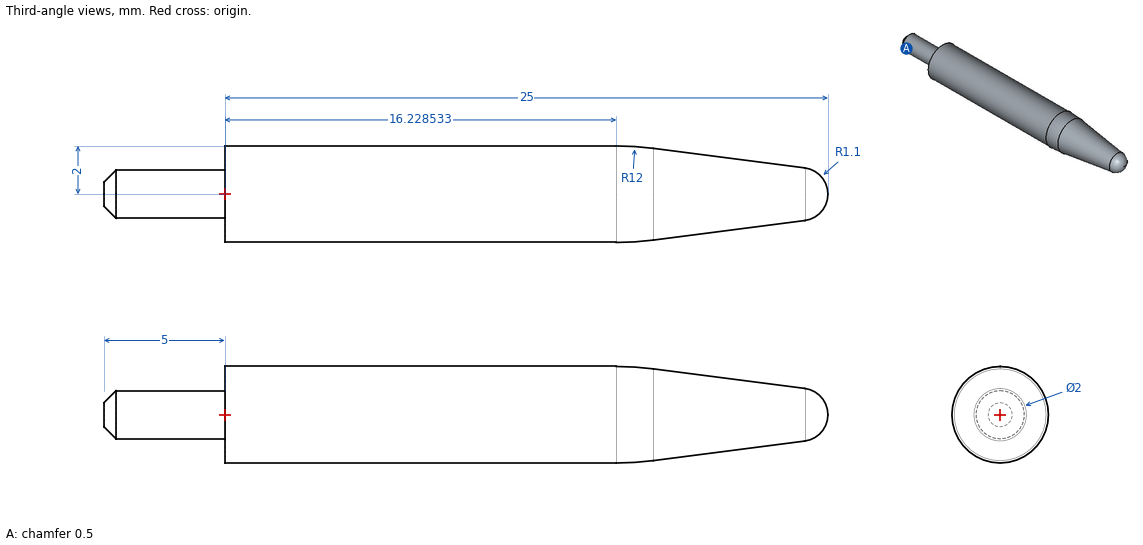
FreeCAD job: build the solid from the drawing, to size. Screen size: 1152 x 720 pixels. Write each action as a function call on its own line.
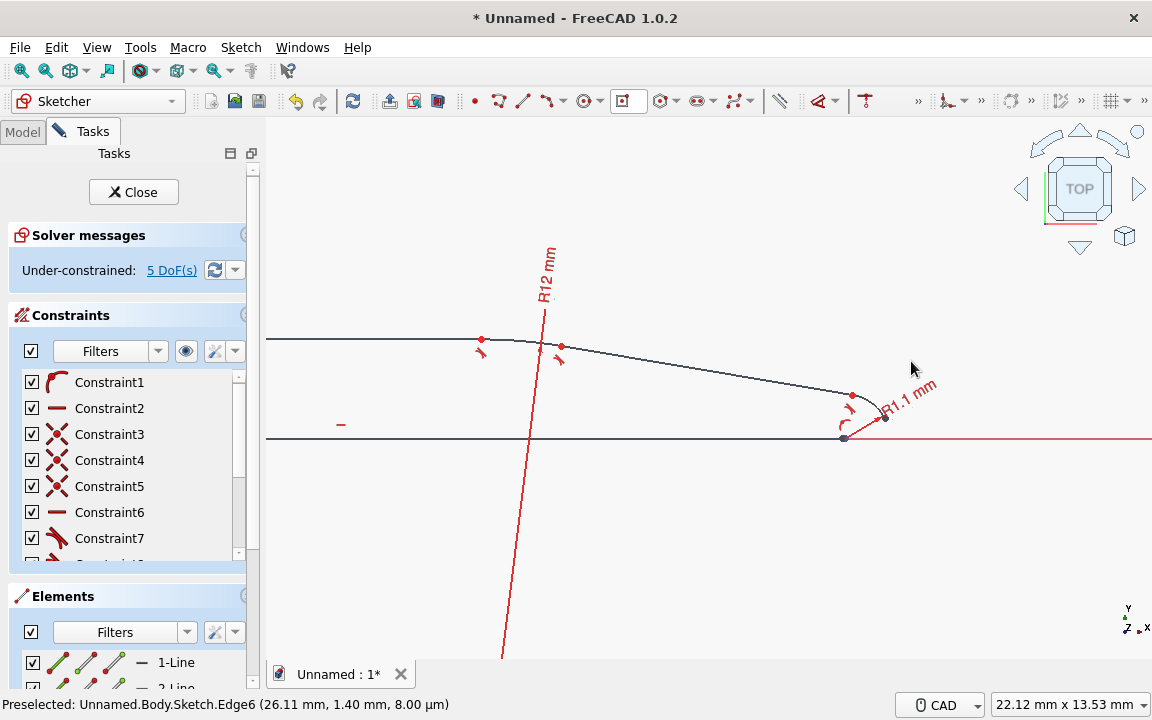
click(885, 419)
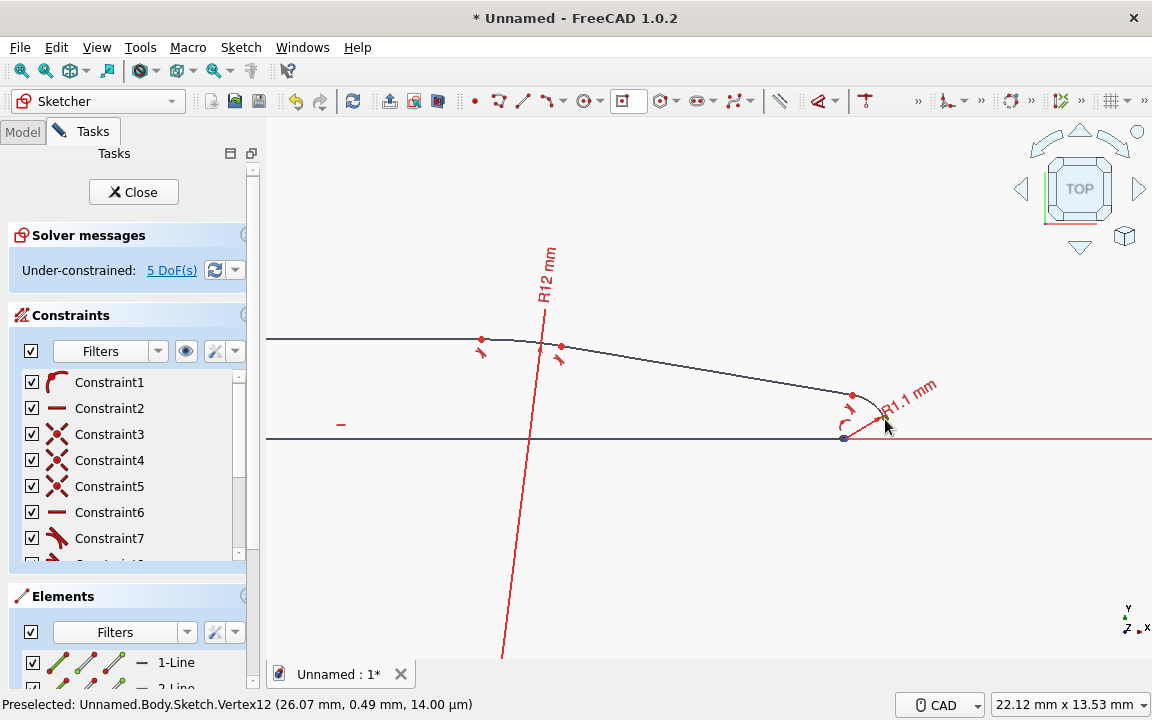
click(938, 439)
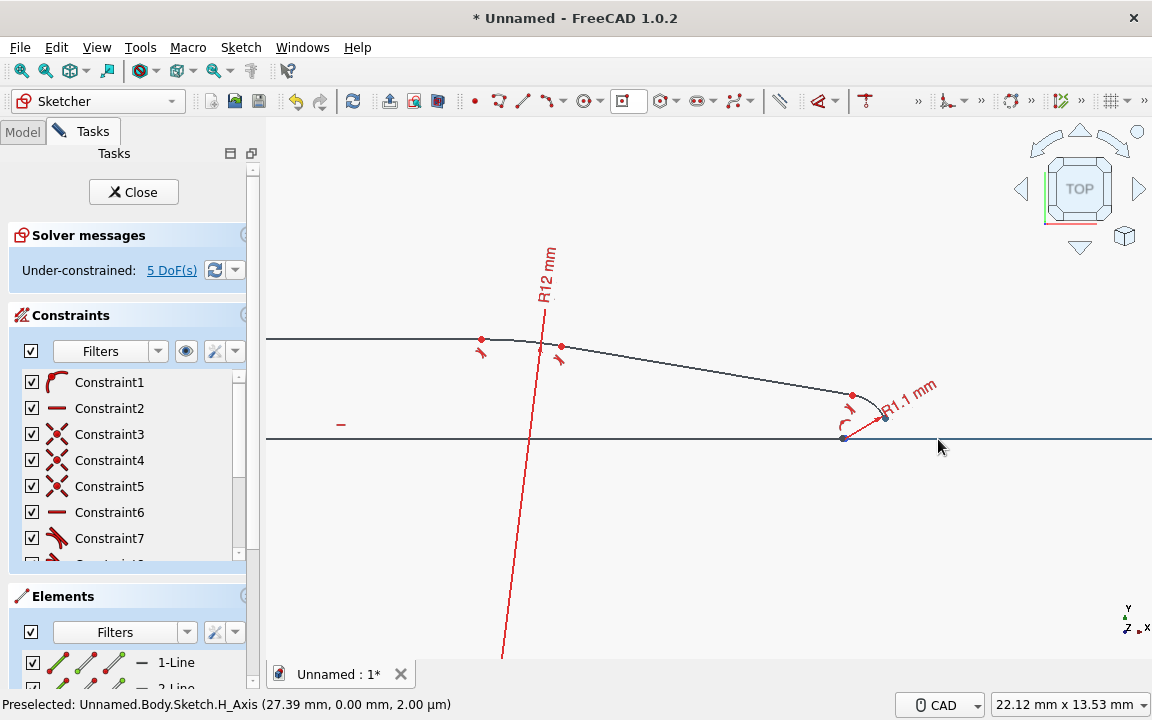
key(c)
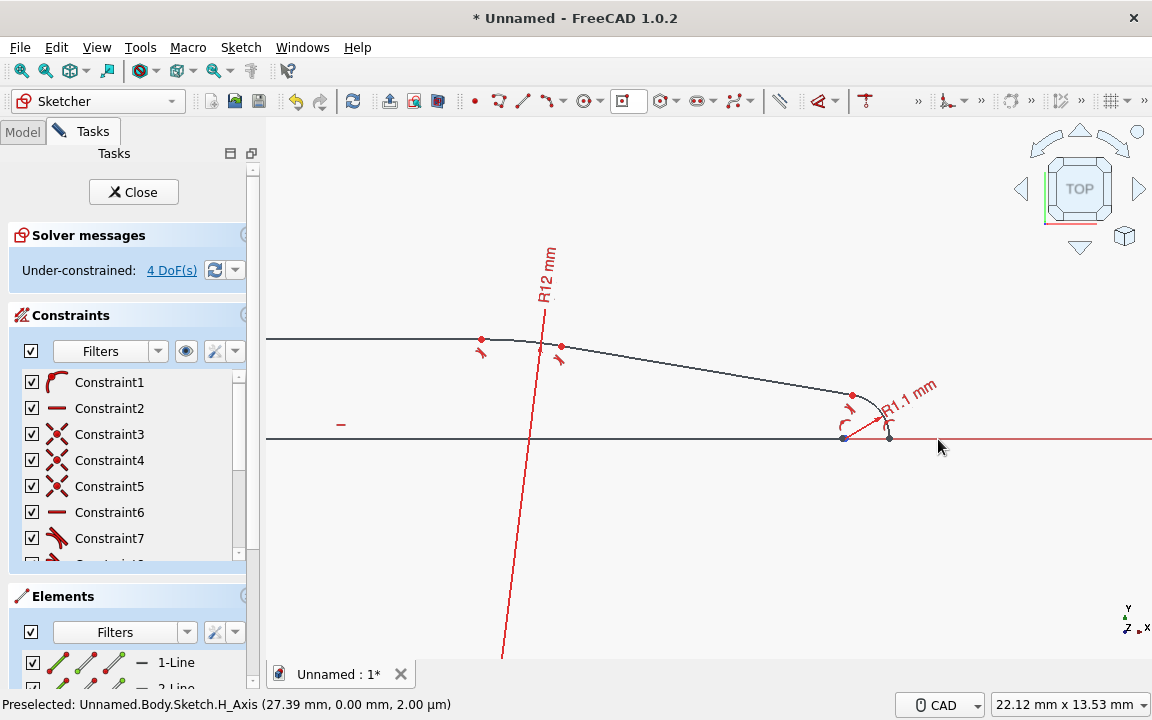
key(d)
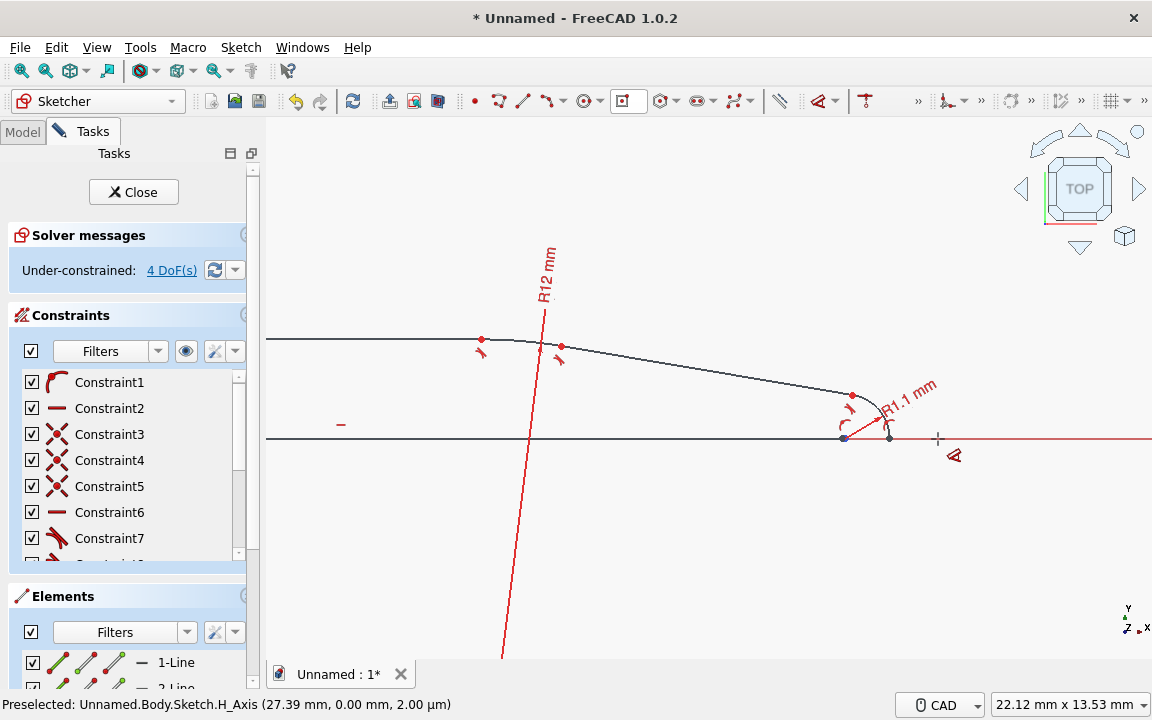
scroll(884, 379, down, 4)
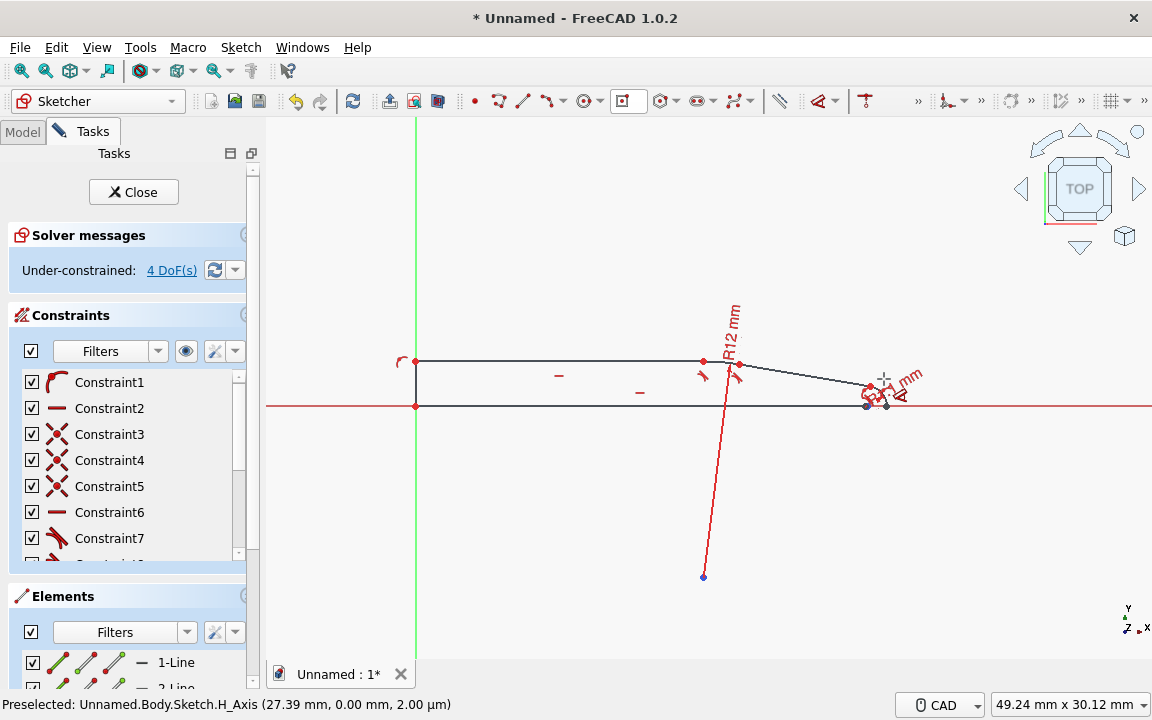
click(416, 375)
click(382, 384)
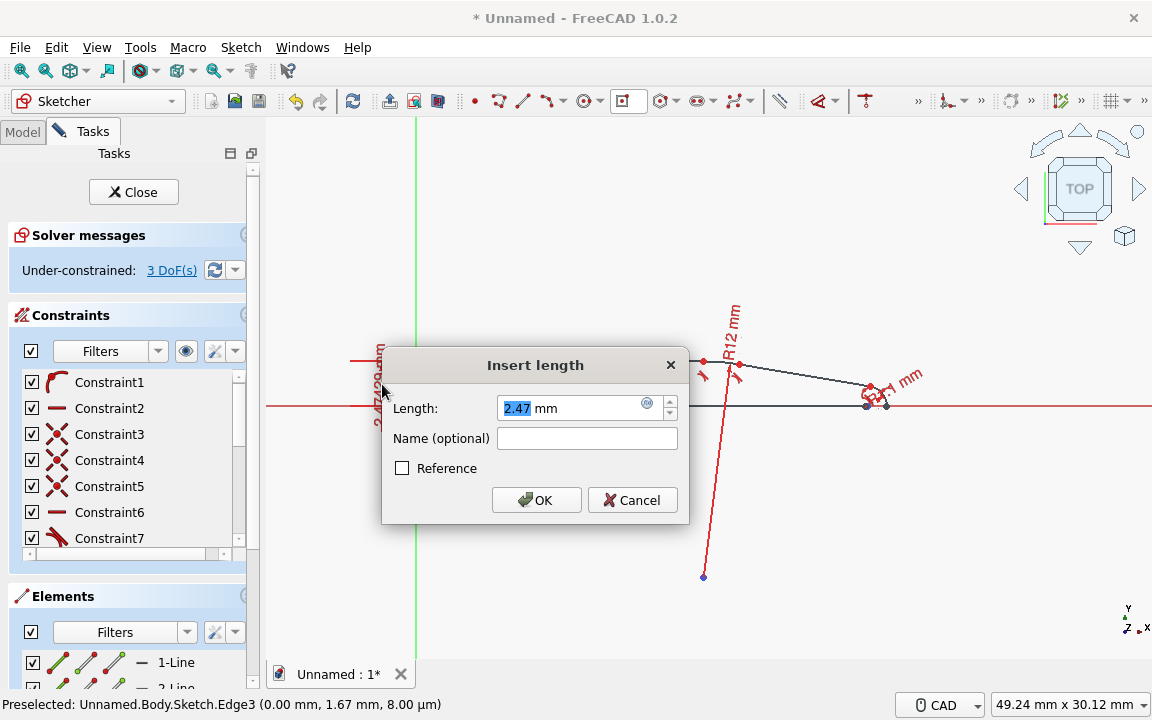
text(2)
key(Return)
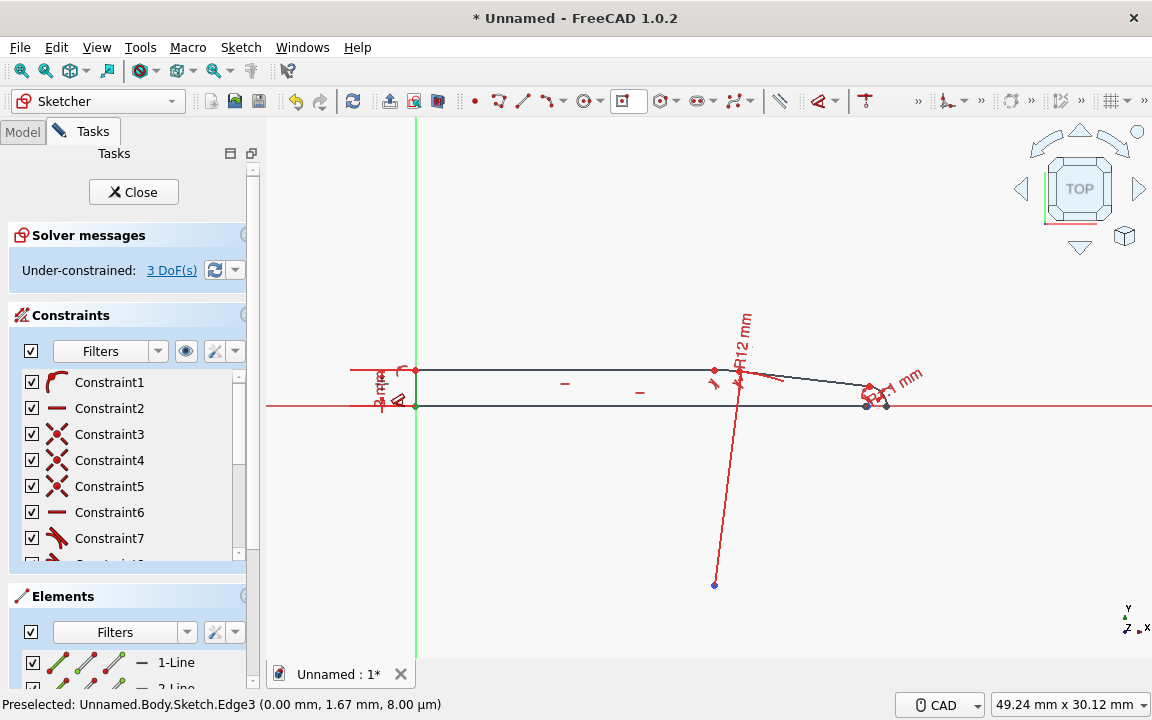
click(551, 406)
click(641, 440)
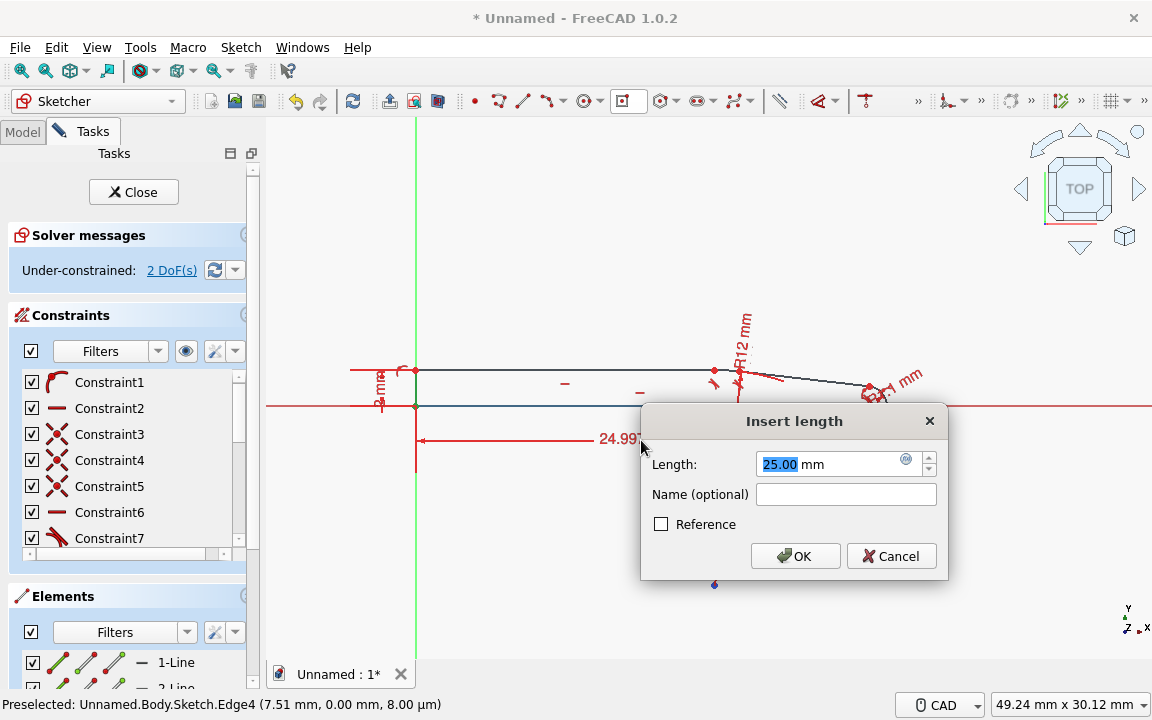
text(25)
key(Return)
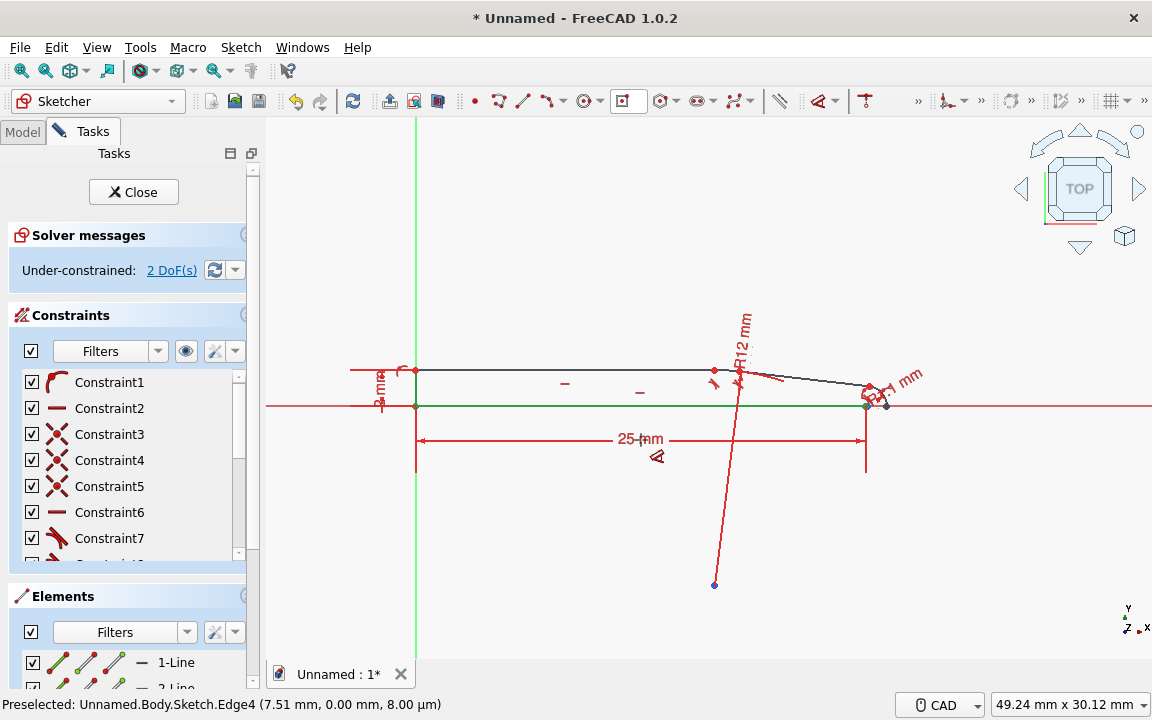
click(887, 406)
click(543, 440)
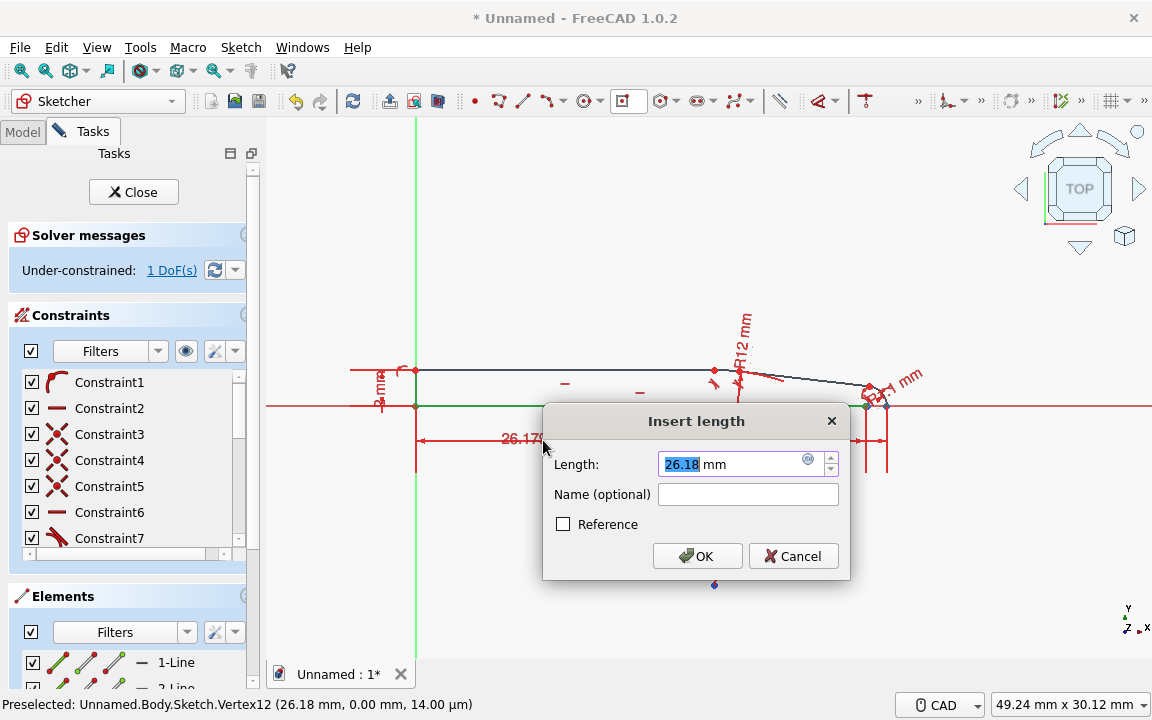
text(25)
key(Return)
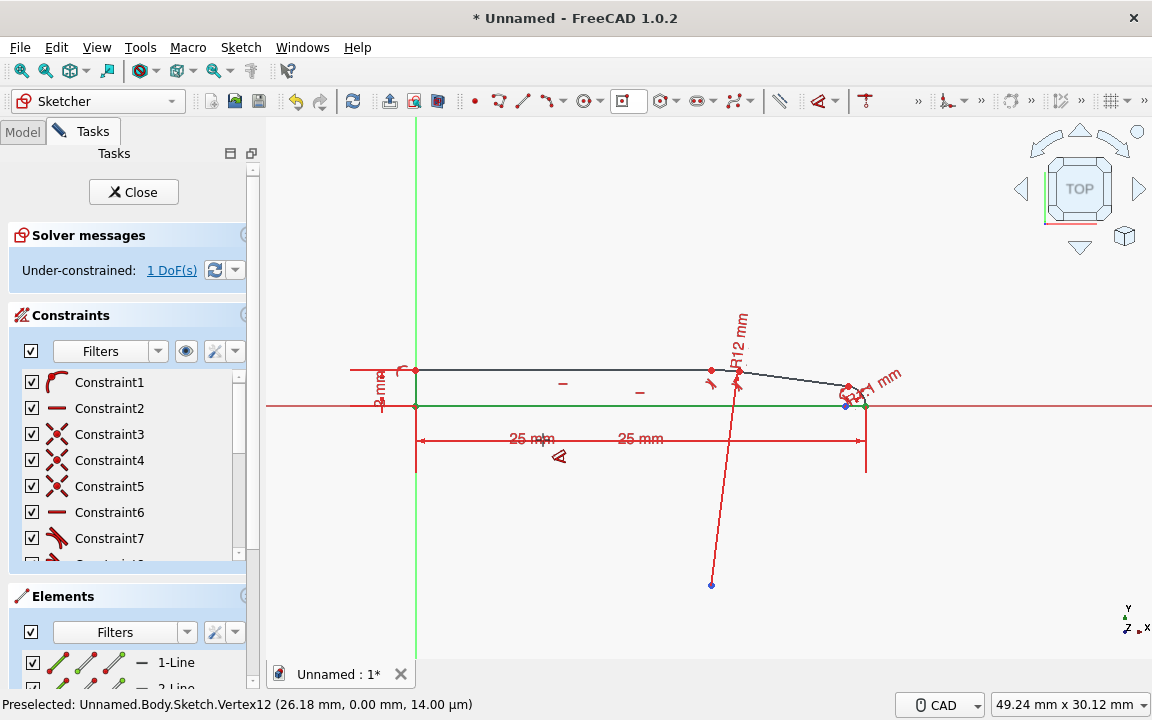
click(623, 370)
click(563, 336)